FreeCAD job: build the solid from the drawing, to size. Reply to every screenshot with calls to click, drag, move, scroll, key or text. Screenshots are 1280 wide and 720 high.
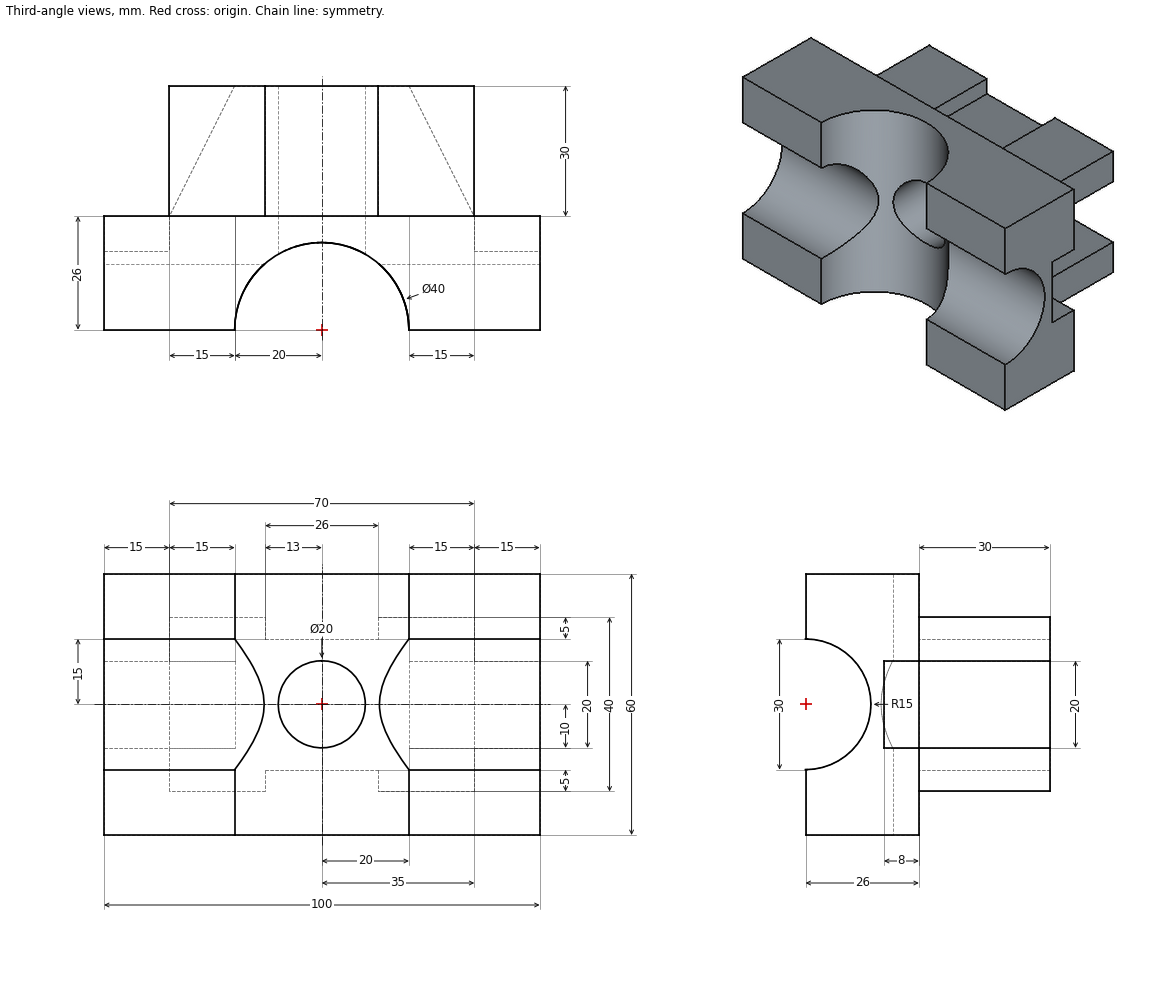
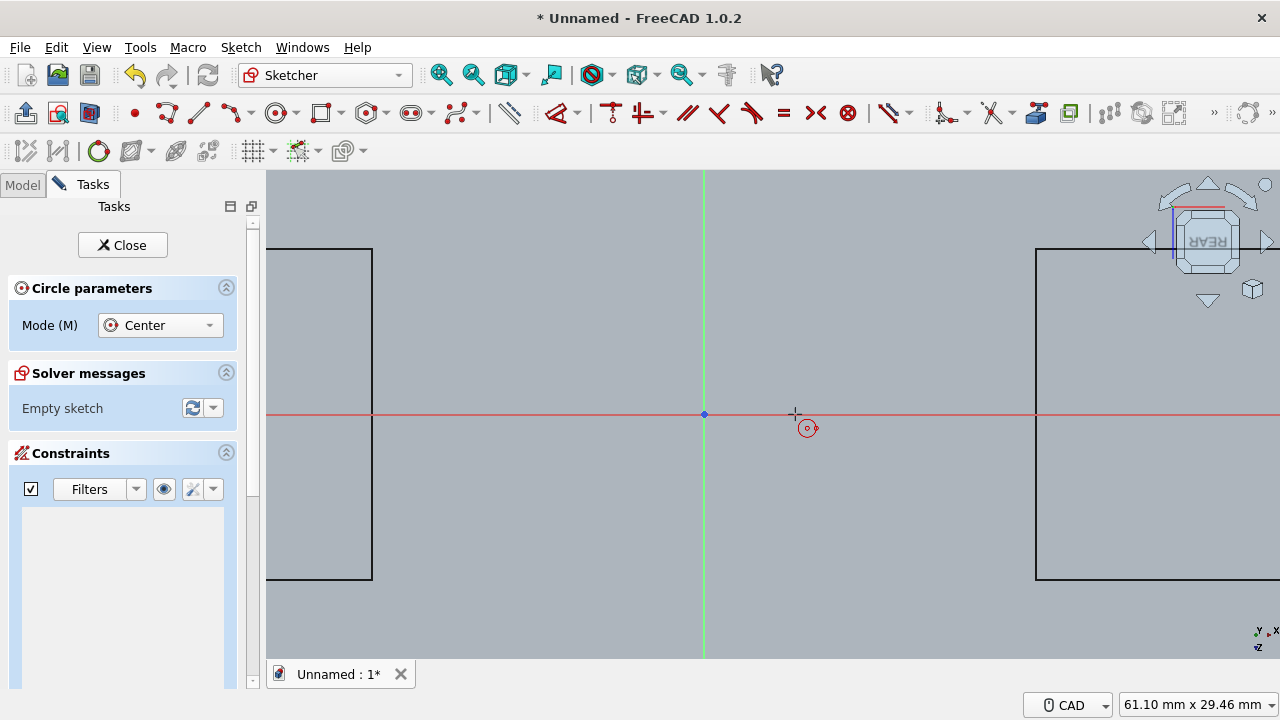
click(704, 414)
move(822, 297)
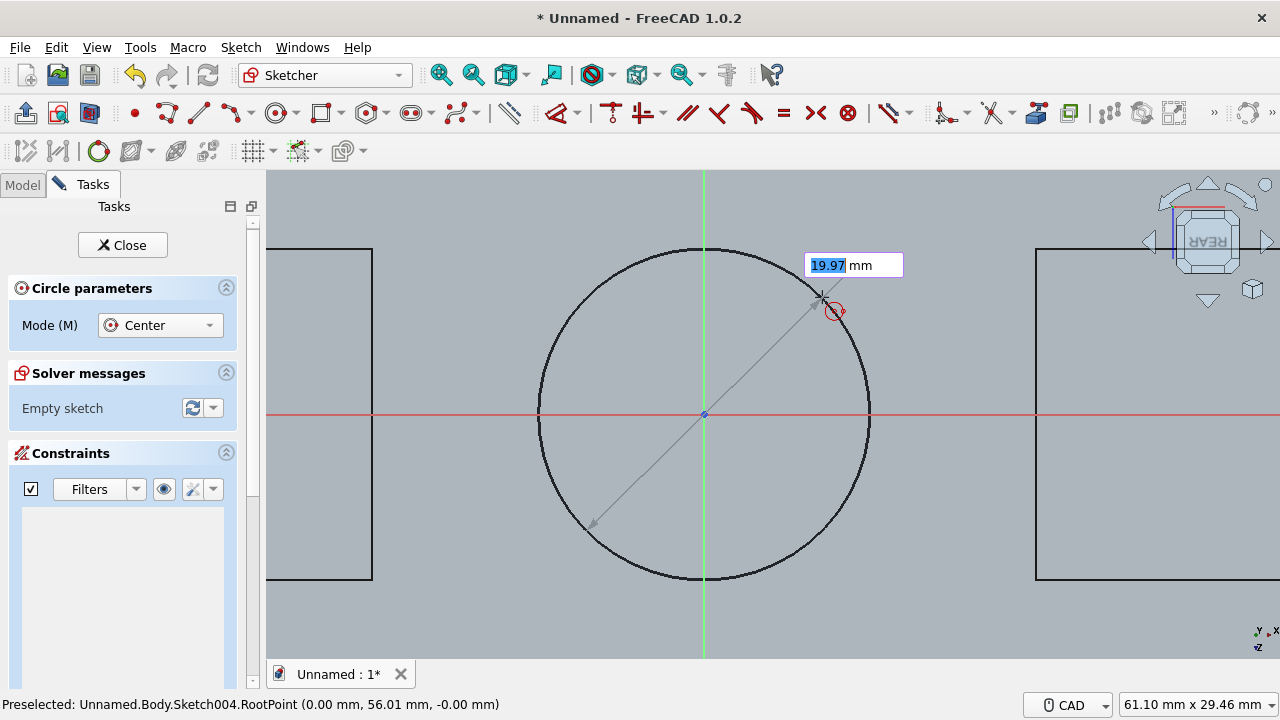
text(20)
key(Return)
key(Escape)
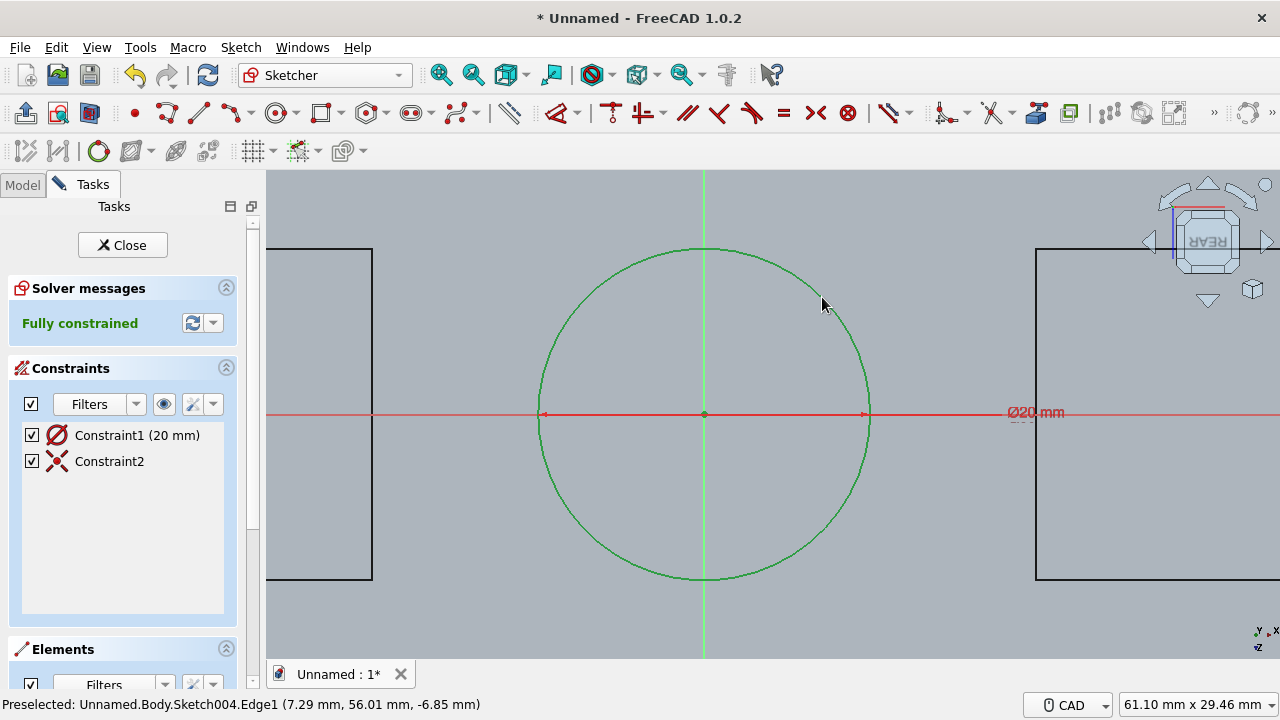
click(123, 245)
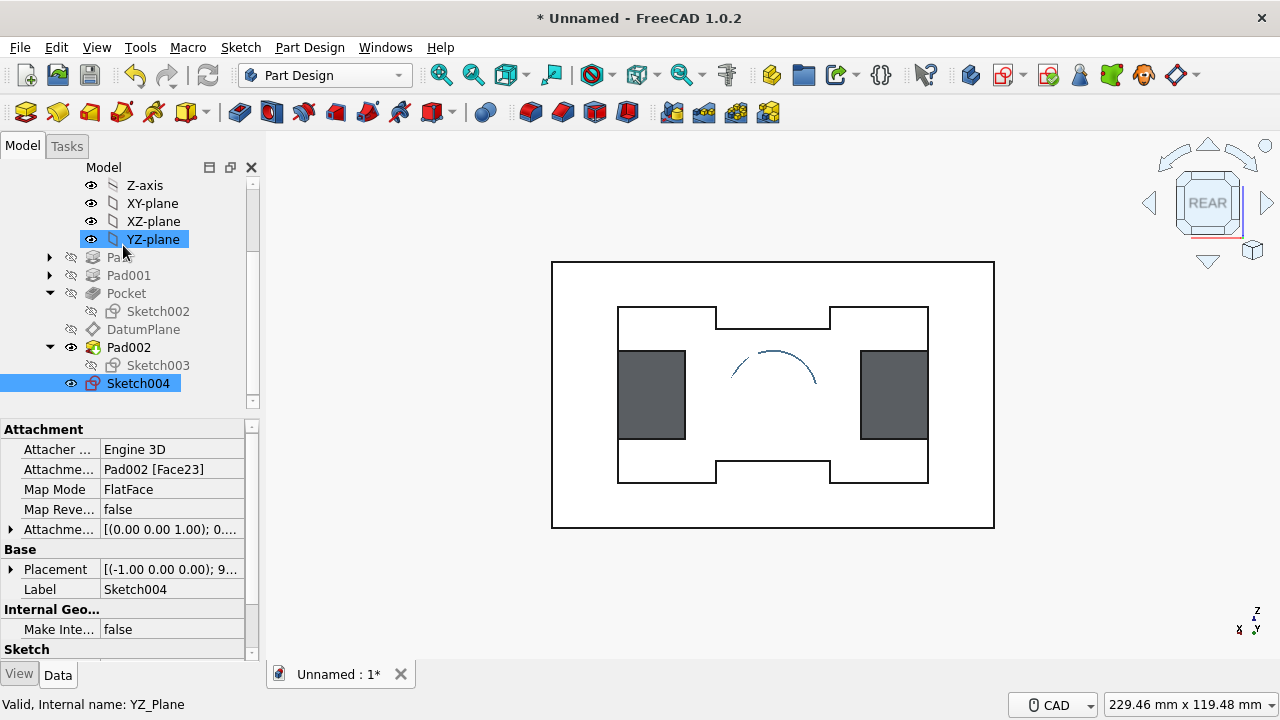
click(240, 112)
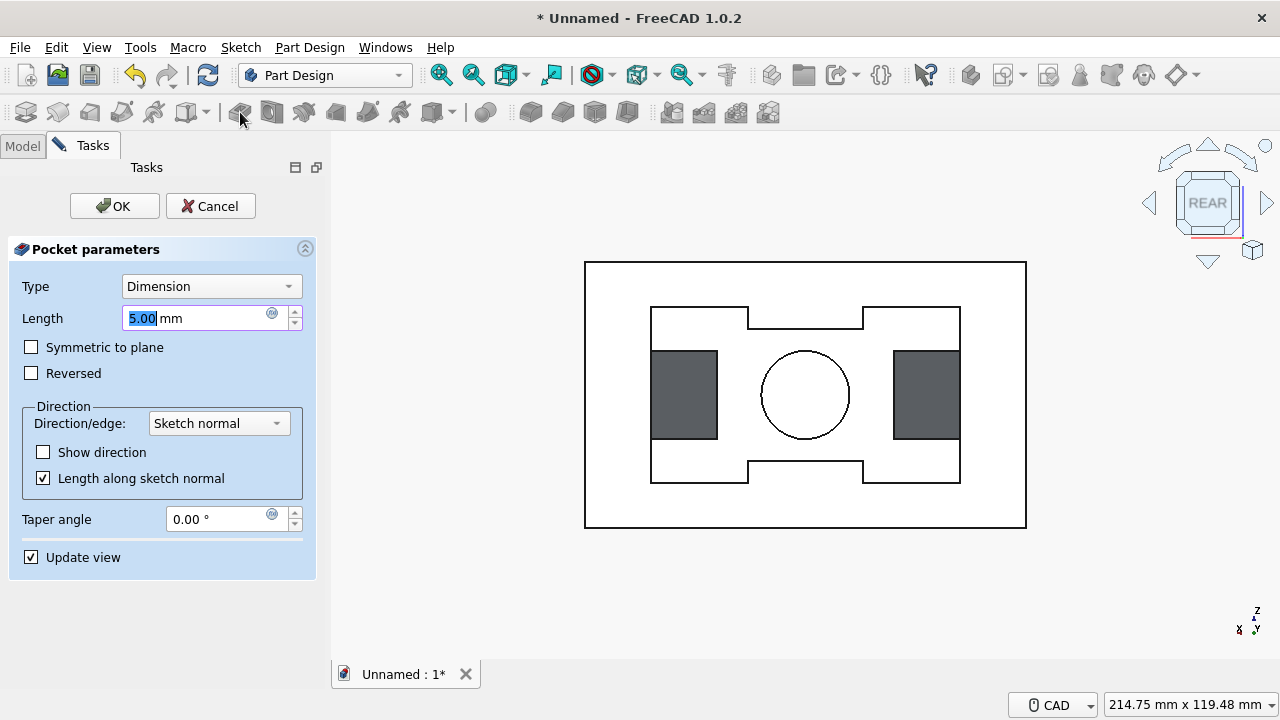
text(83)
key(Tab)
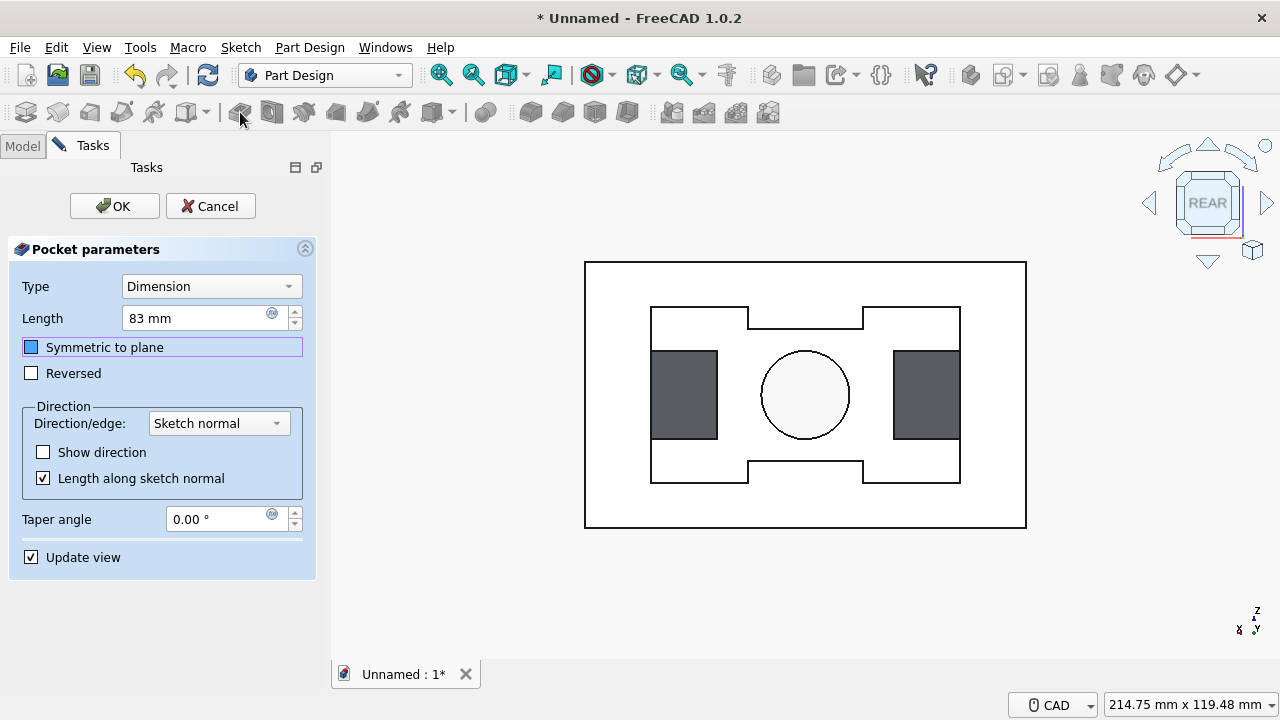
click(115, 206)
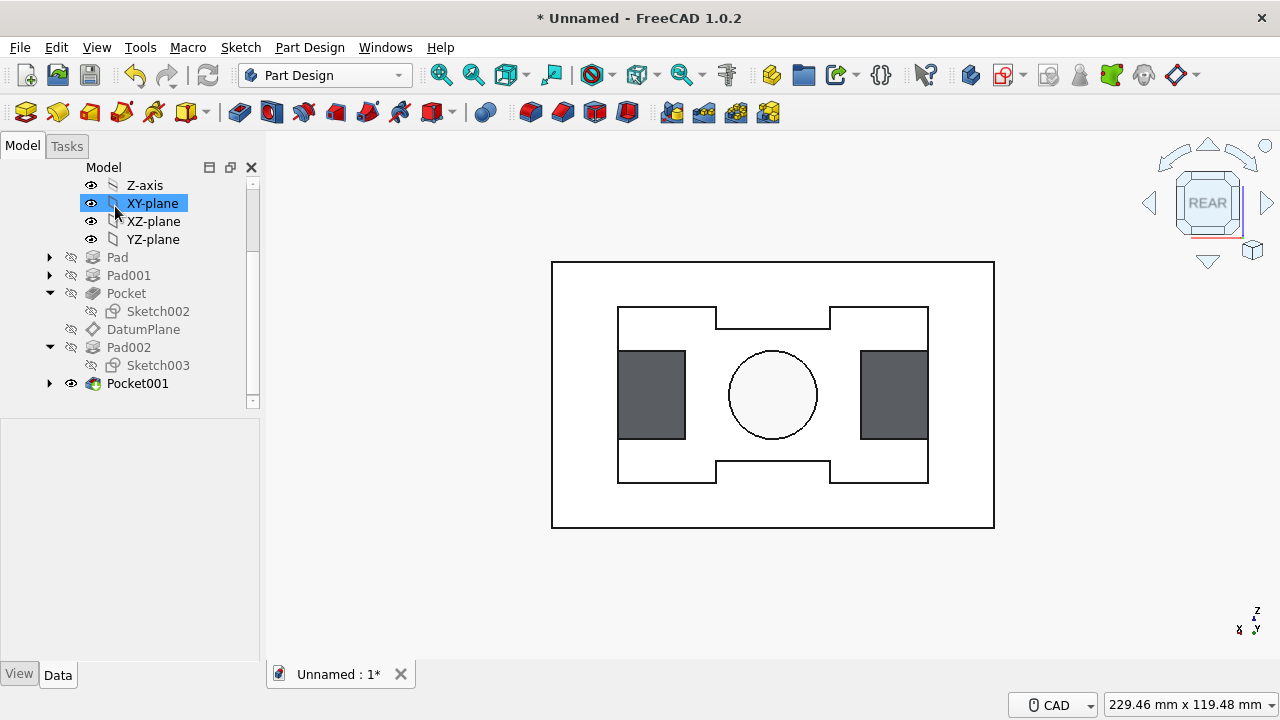
click(962, 318)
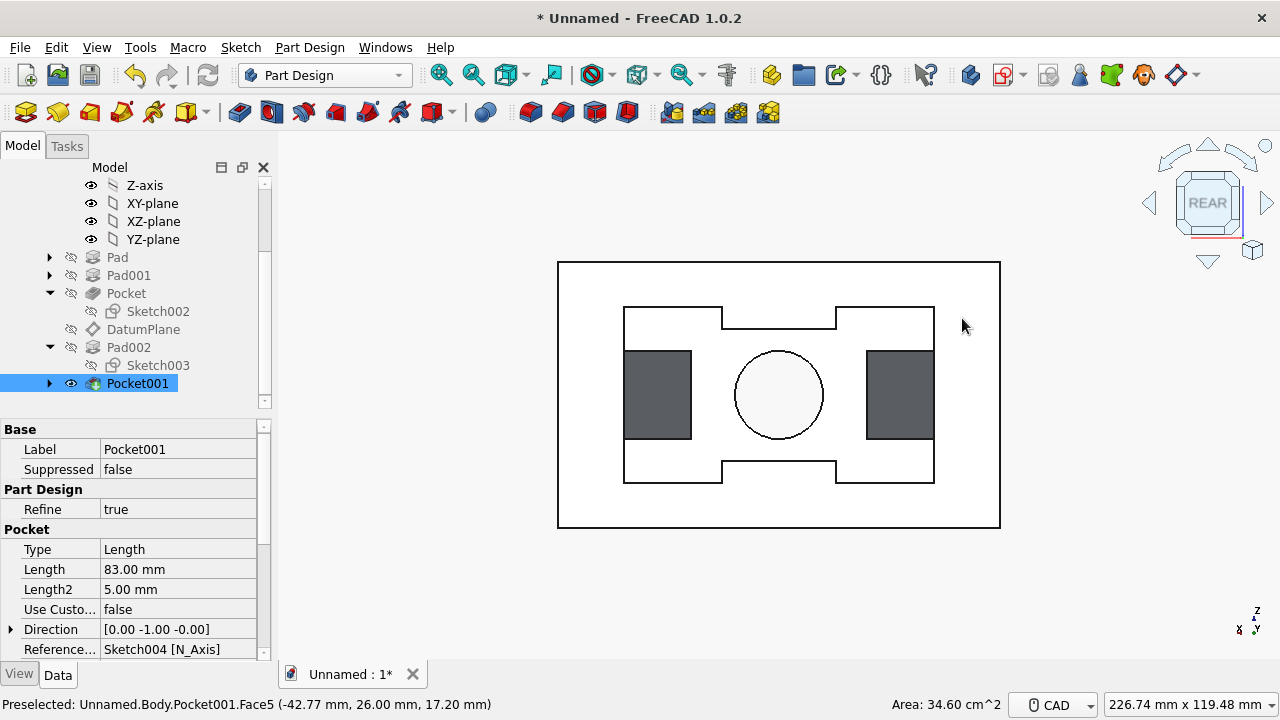
click(1004, 76)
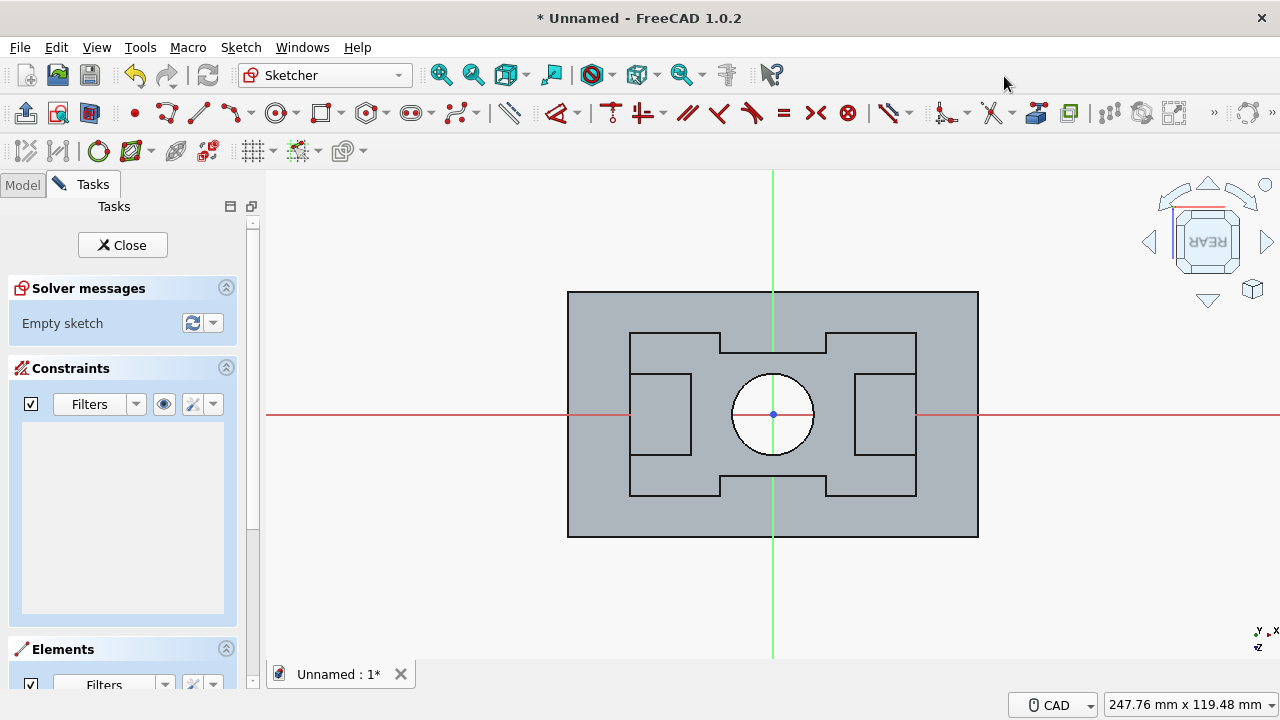
scroll(912, 414, up, 2)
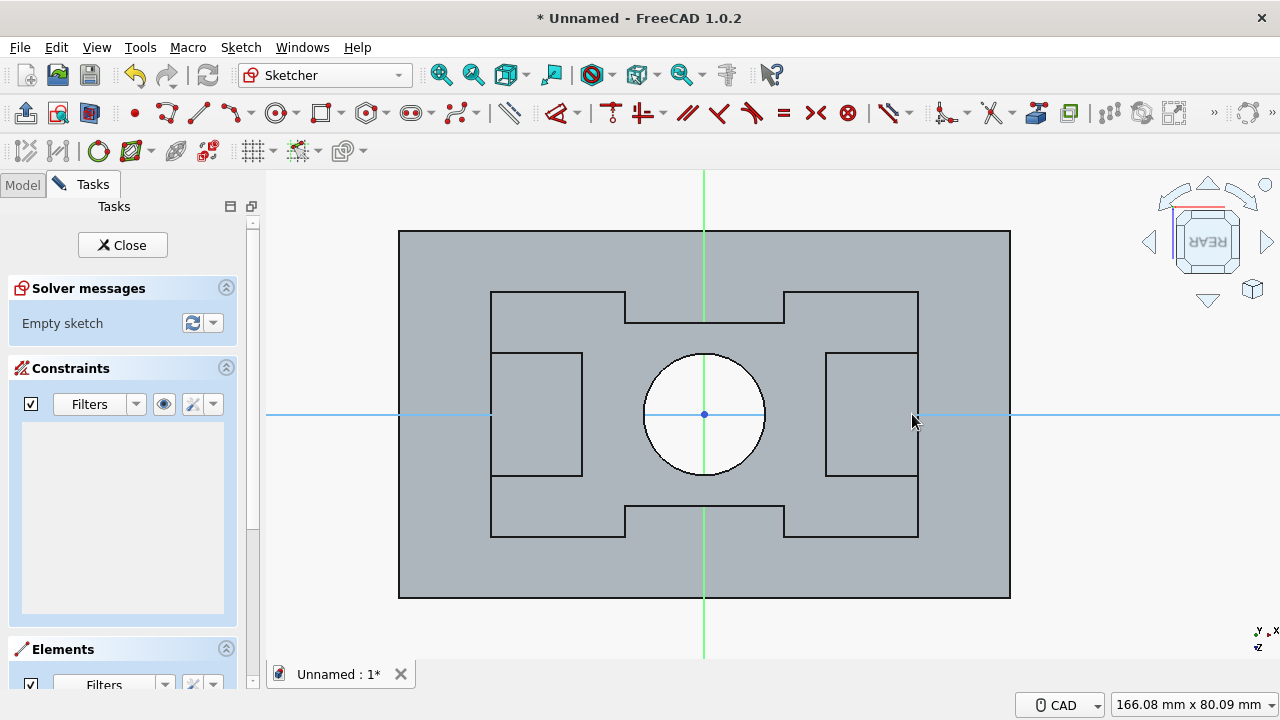
key(g)
key(r)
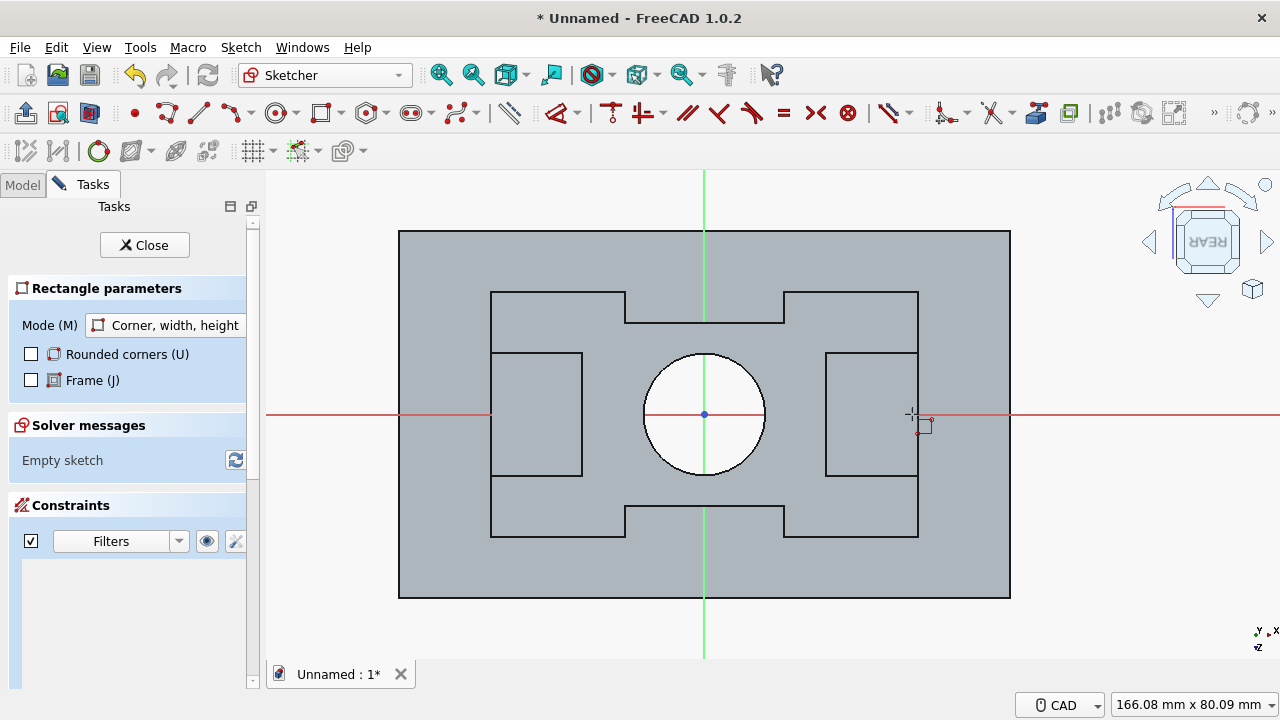
click(918, 353)
move(1010, 476)